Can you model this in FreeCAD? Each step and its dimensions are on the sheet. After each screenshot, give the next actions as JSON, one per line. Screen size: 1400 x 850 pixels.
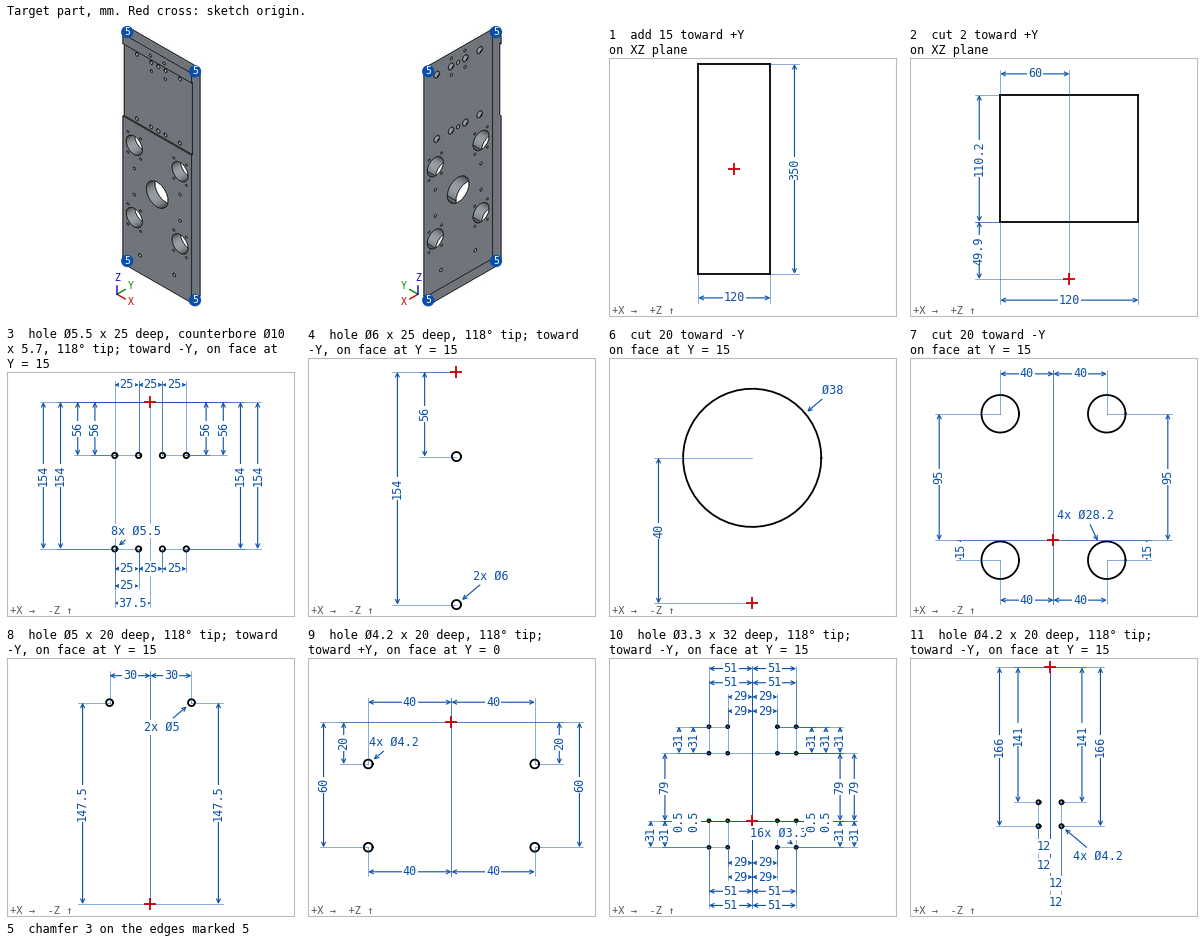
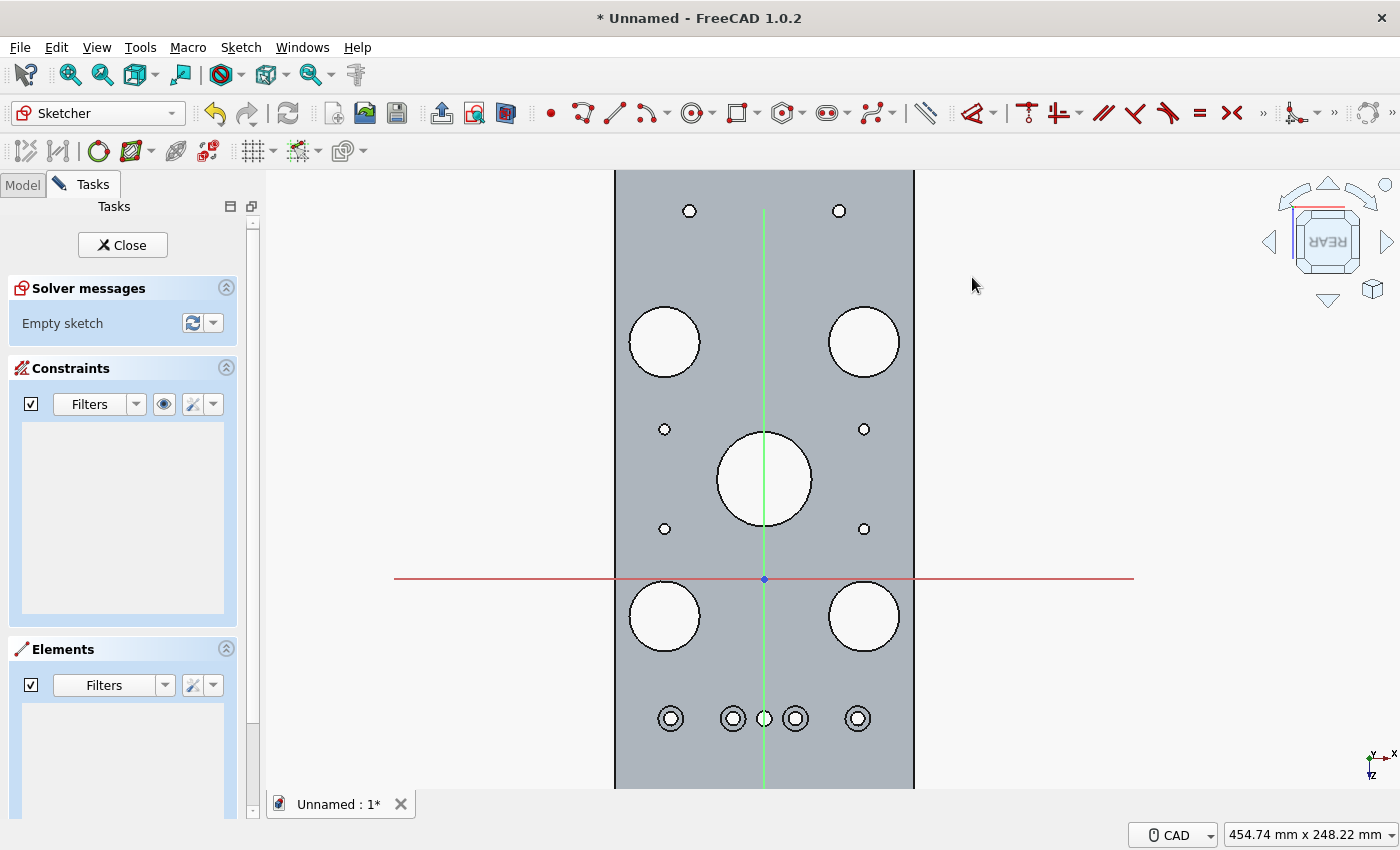
{"action": "left_click", "coordinate": [692, 114]}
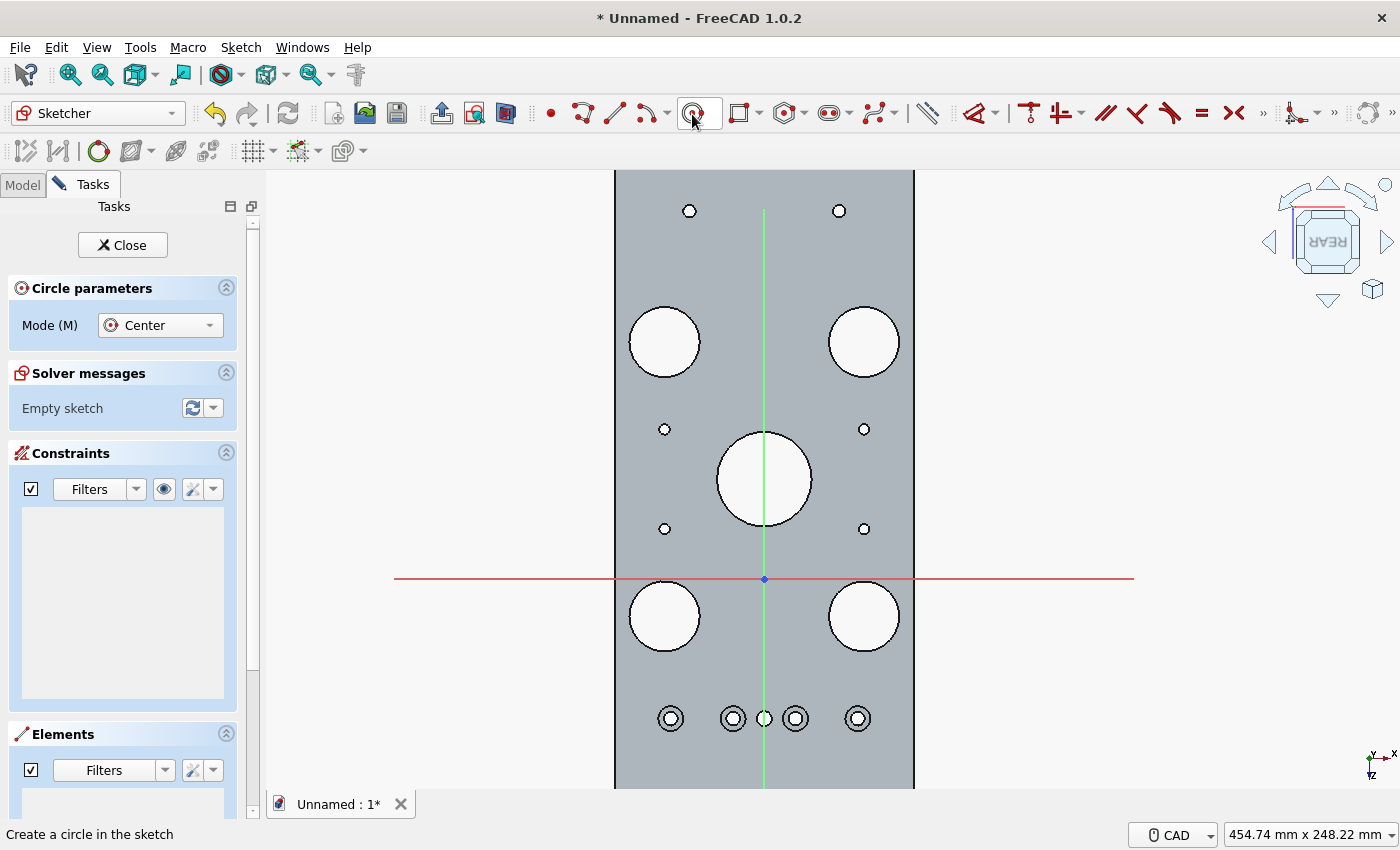
{"action": "scroll", "coordinate": [892, 655], "scroll_direction": "up", "scroll_amount": 9}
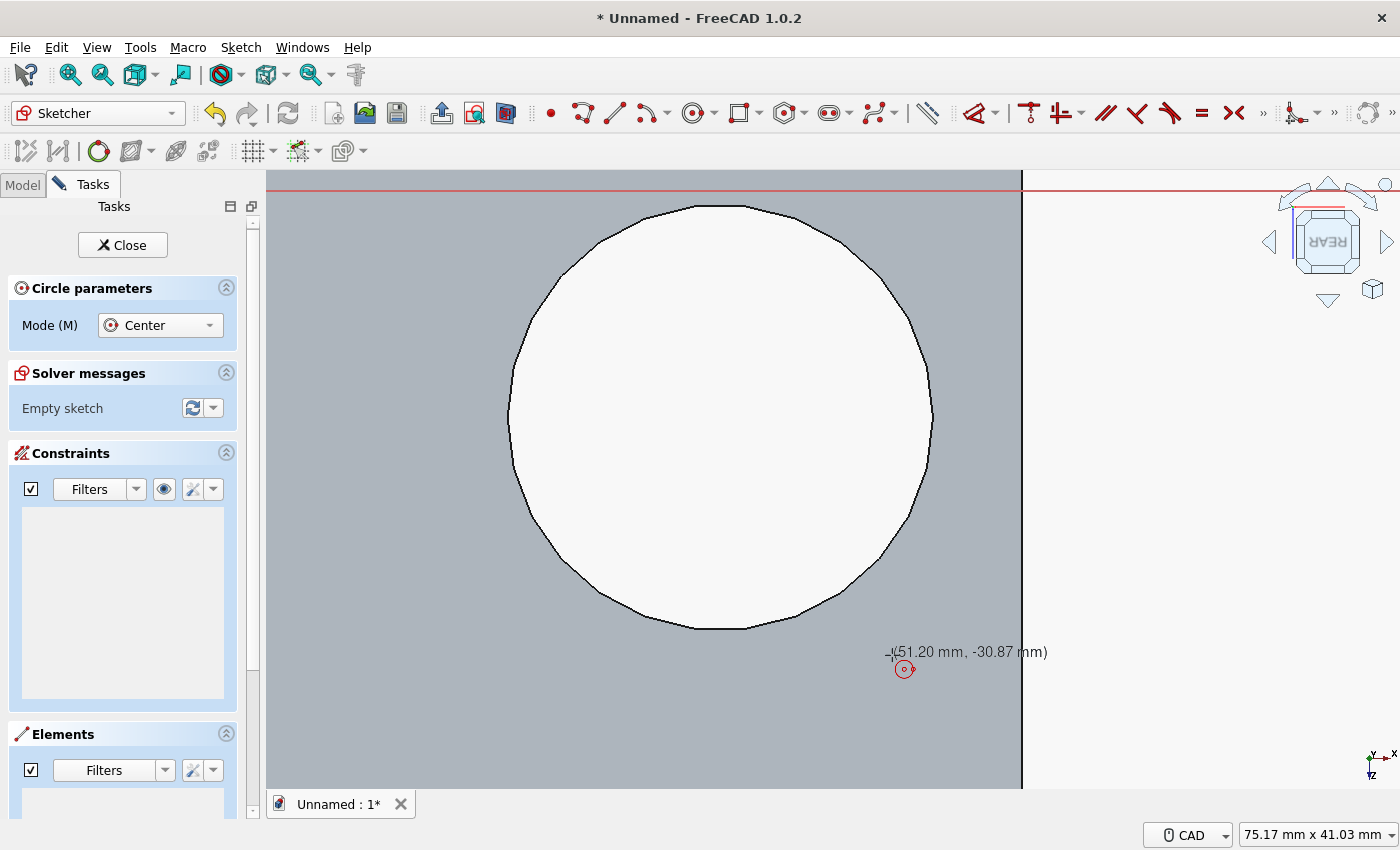
{"action": "scroll", "coordinate": [893, 656], "scroll_direction": "down", "scroll_amount": 9}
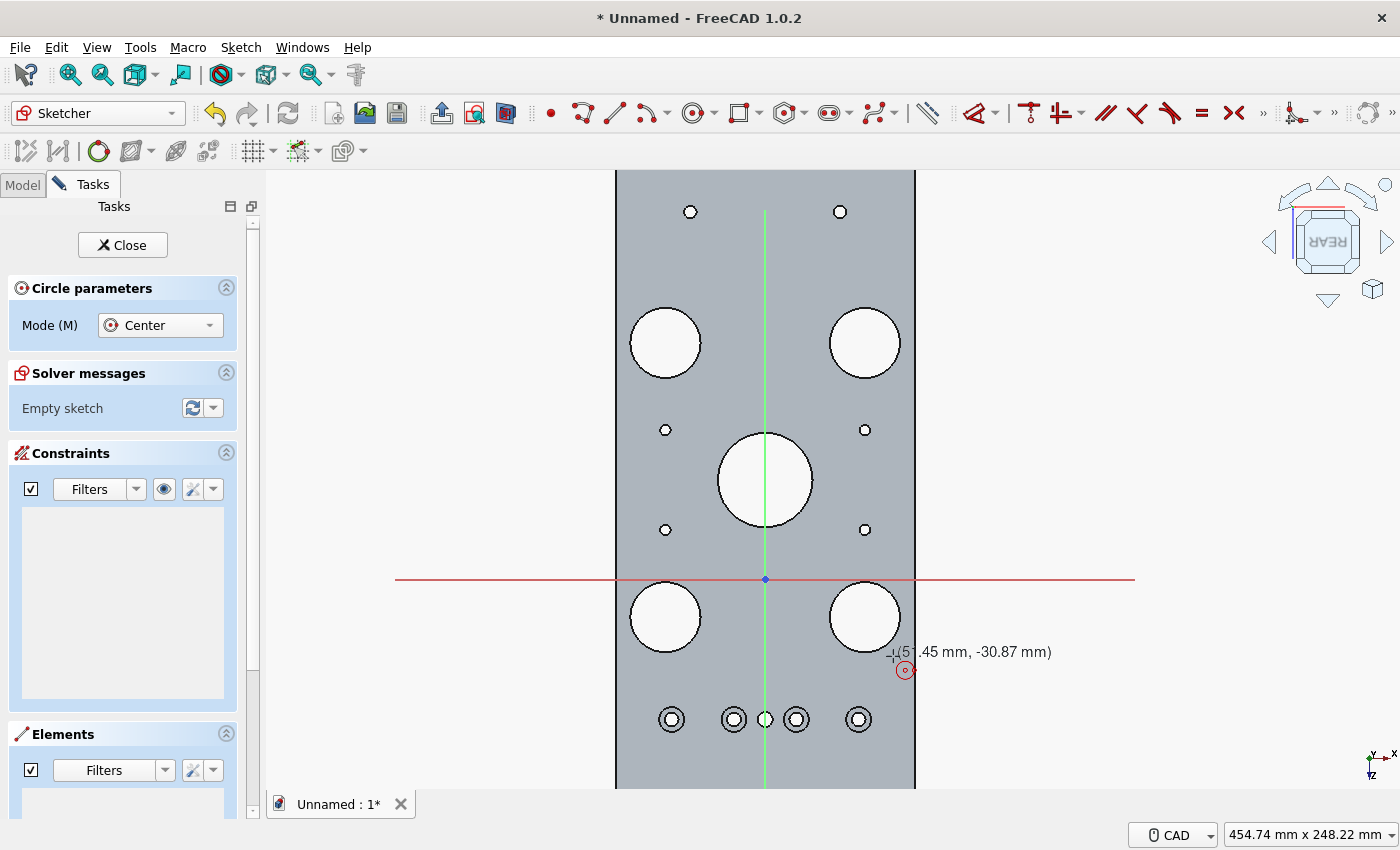
{"action": "left_click", "coordinate": [892, 656]}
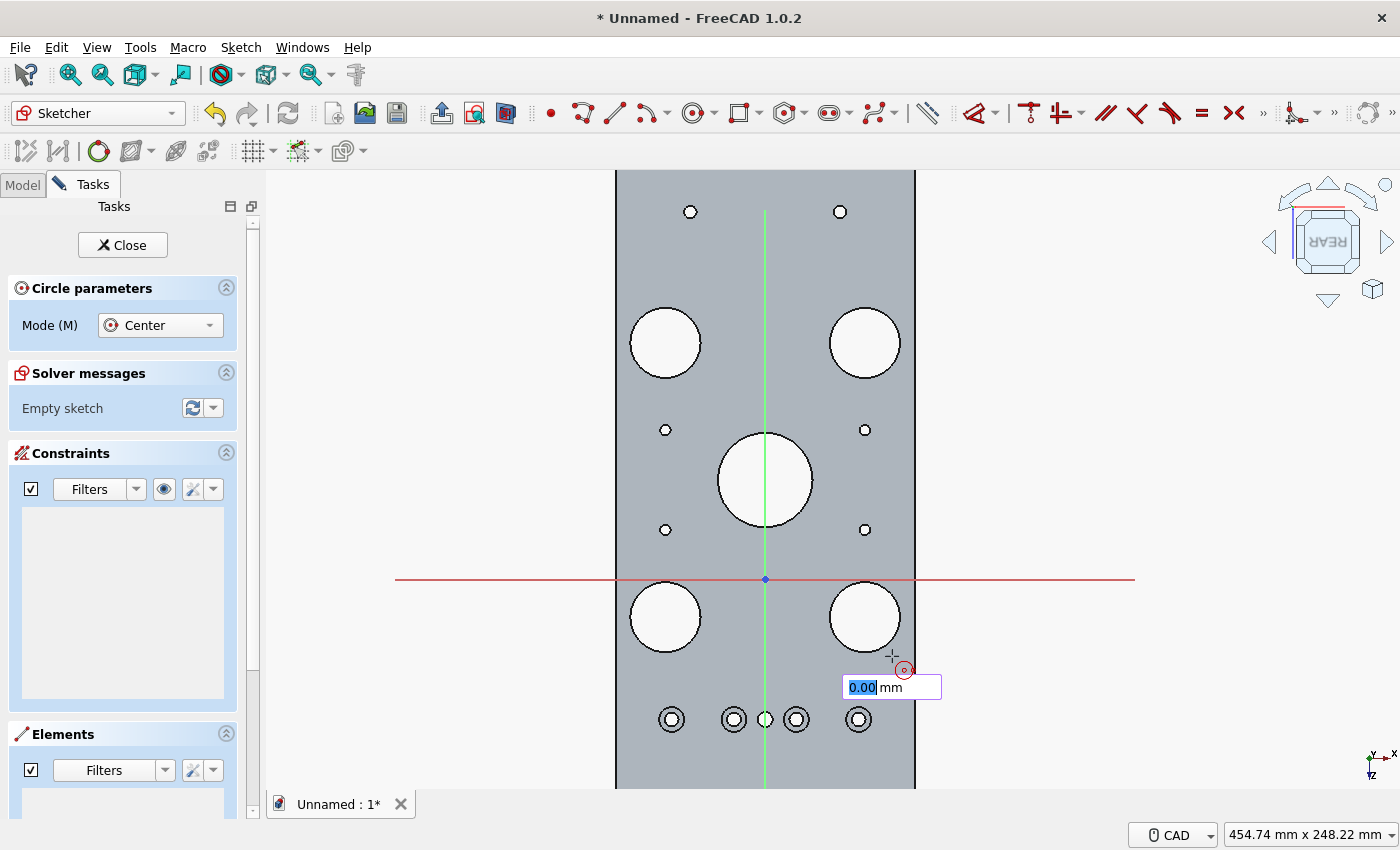
{"action": "scroll", "coordinate": [895, 653], "scroll_direction": "up", "scroll_amount": 7}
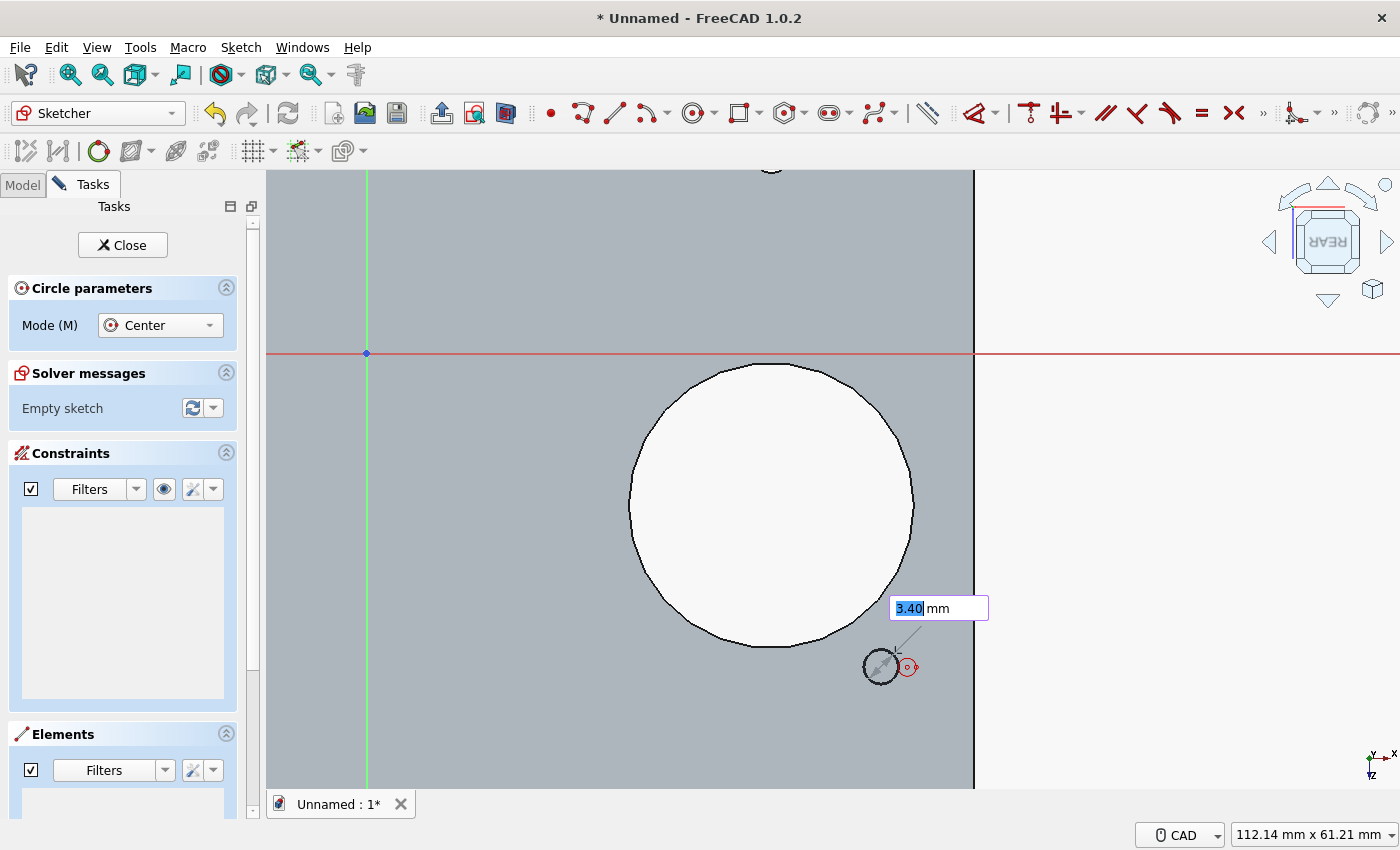
{"action": "left_click", "coordinate": [894, 651]}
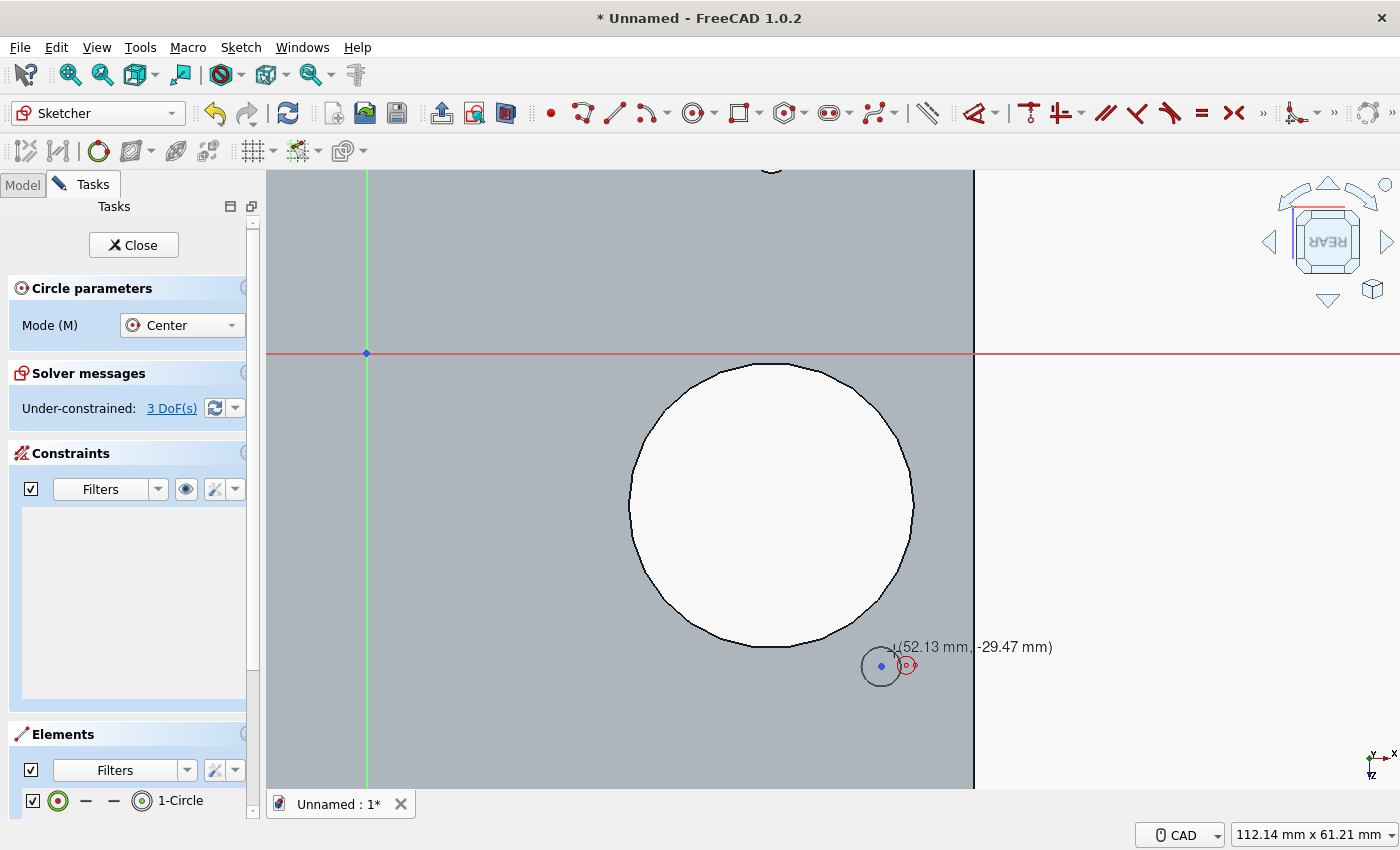
{"action": "scroll", "coordinate": [660, 662], "scroll_direction": "up", "scroll_amount": 2}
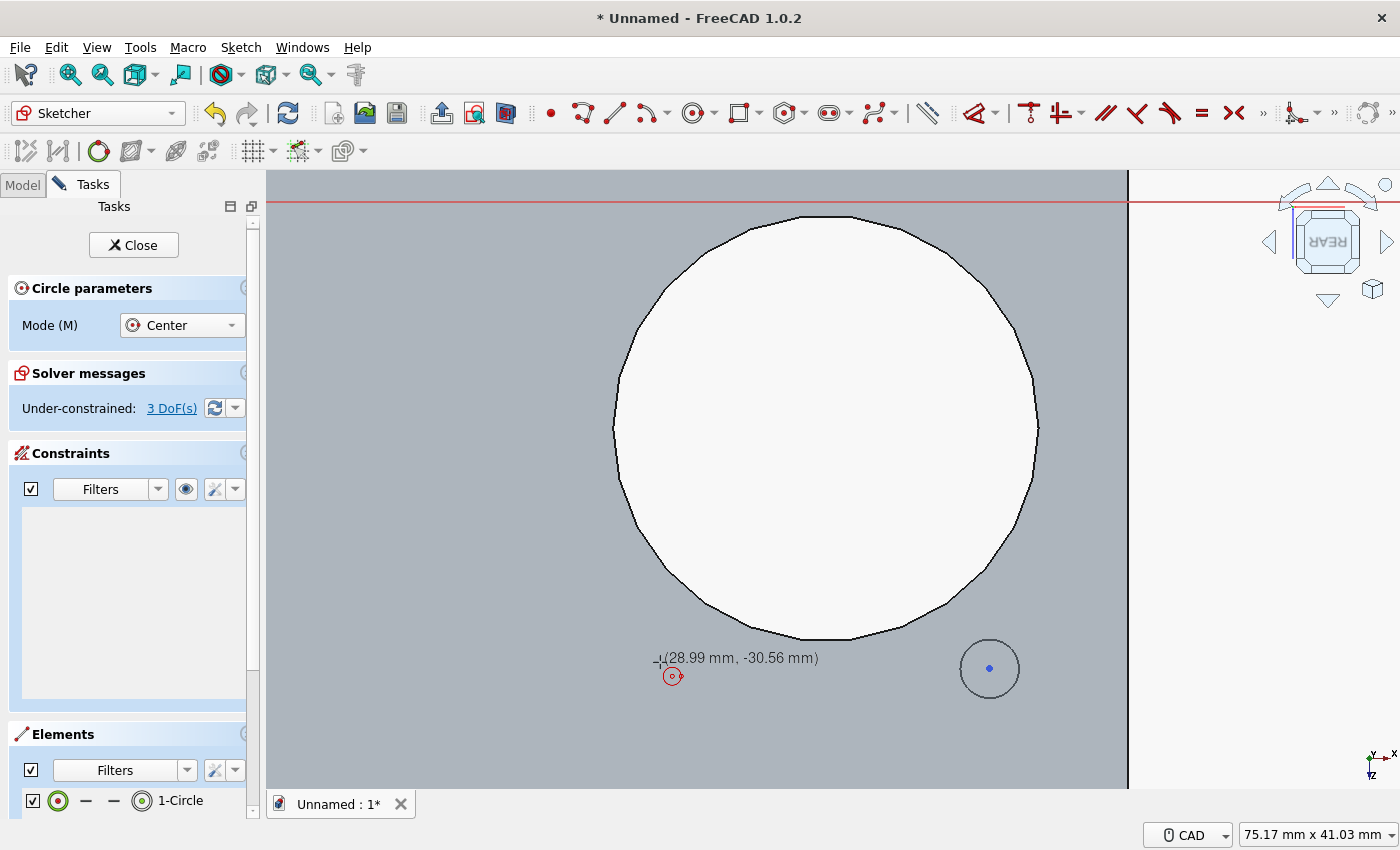
{"action": "scroll", "coordinate": [872, 654], "scroll_direction": "down", "scroll_amount": 9}